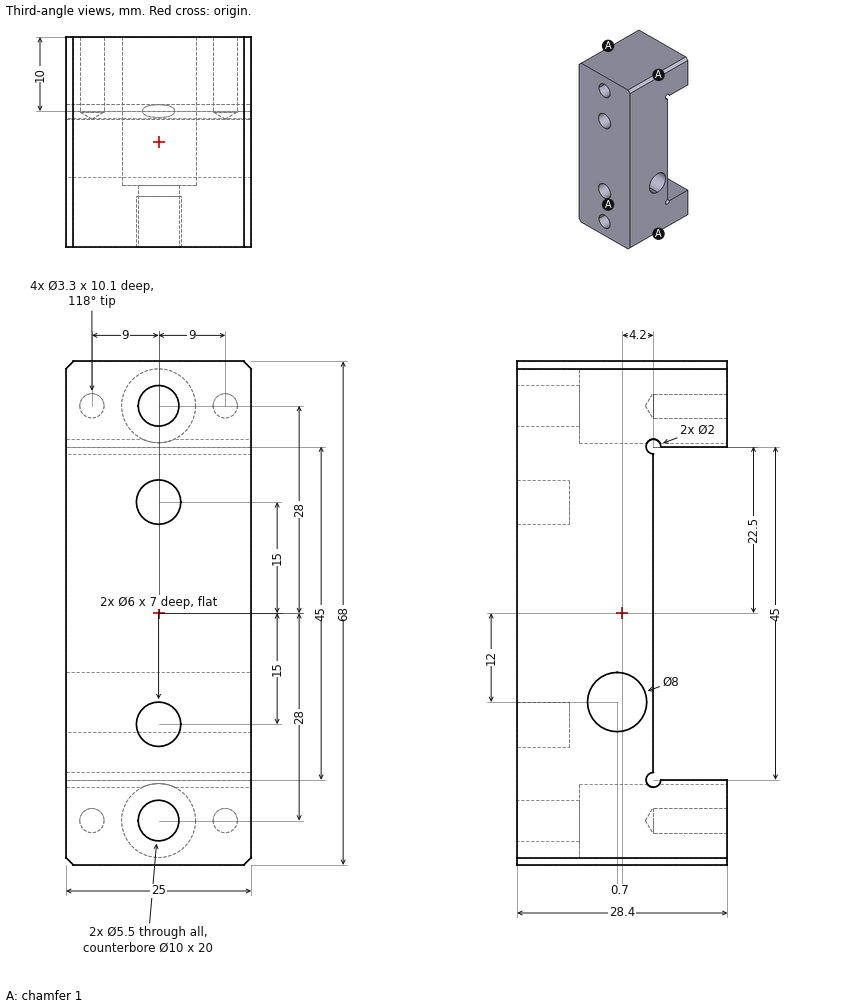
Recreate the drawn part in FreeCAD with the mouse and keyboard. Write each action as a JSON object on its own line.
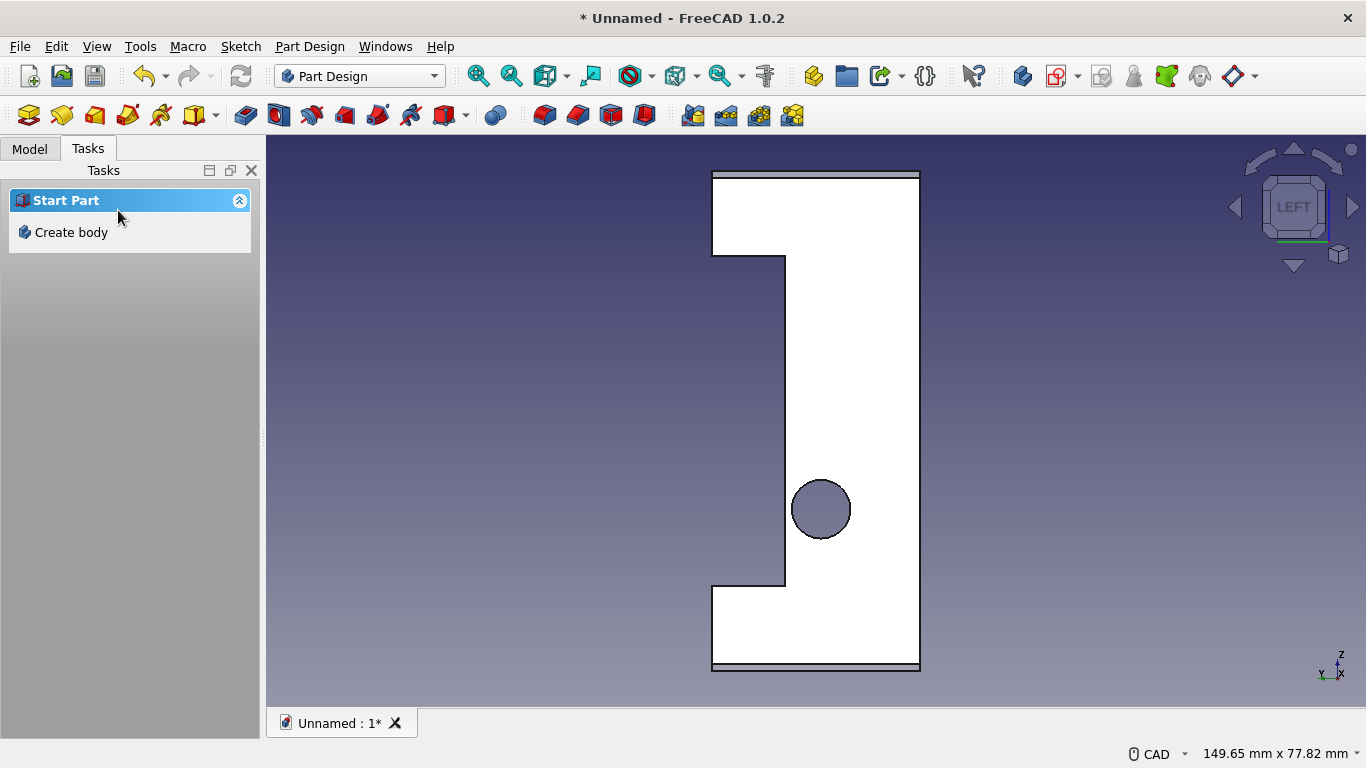
{"action": "key", "text": "0"}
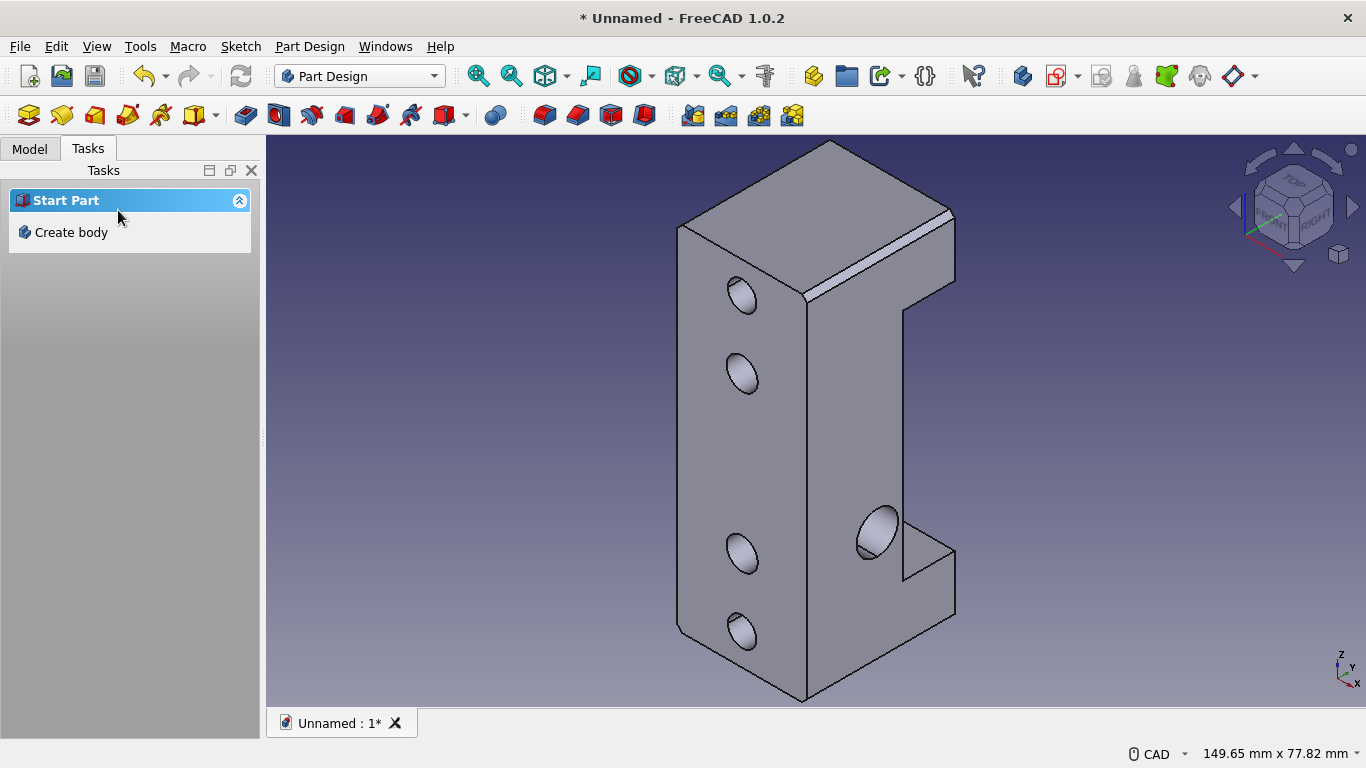
{"action": "left_click", "coordinate": [860, 470]}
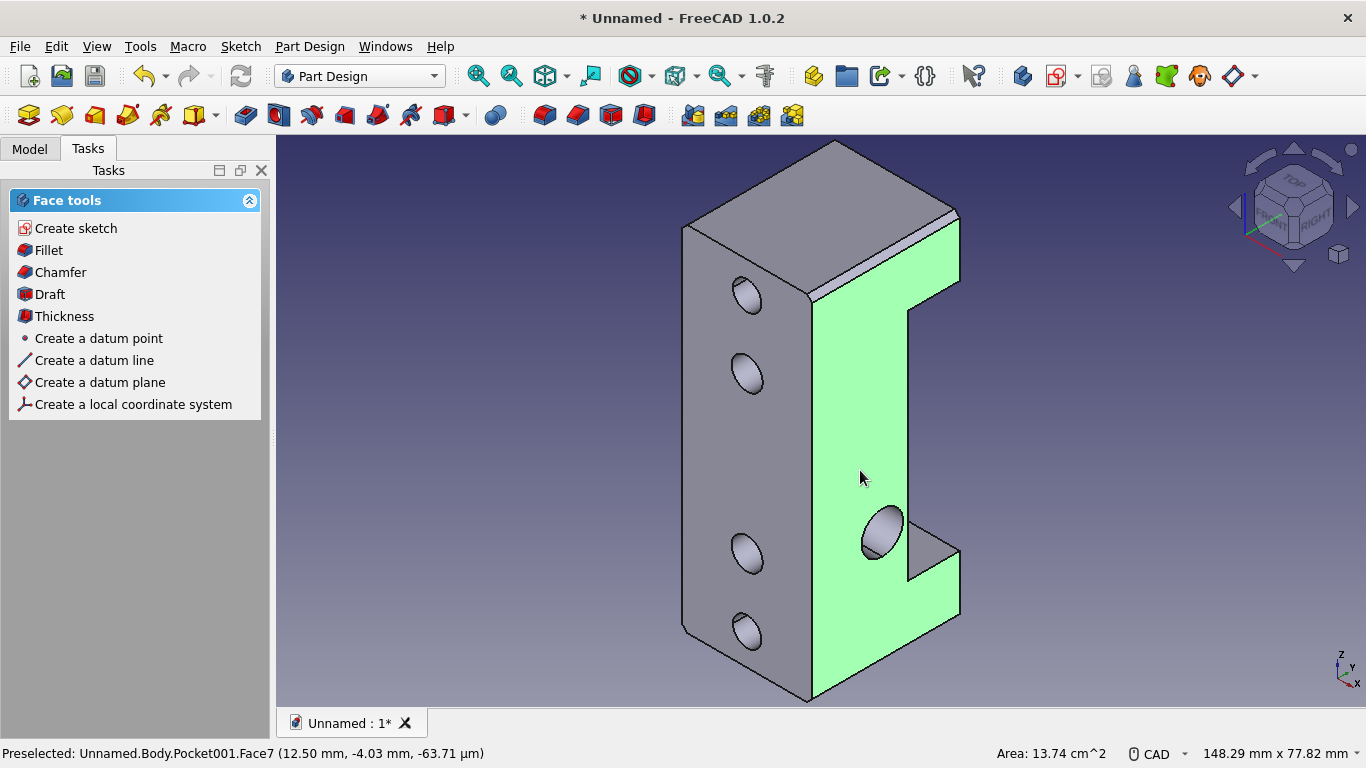
{"action": "left_click", "coordinate": [1056, 76]}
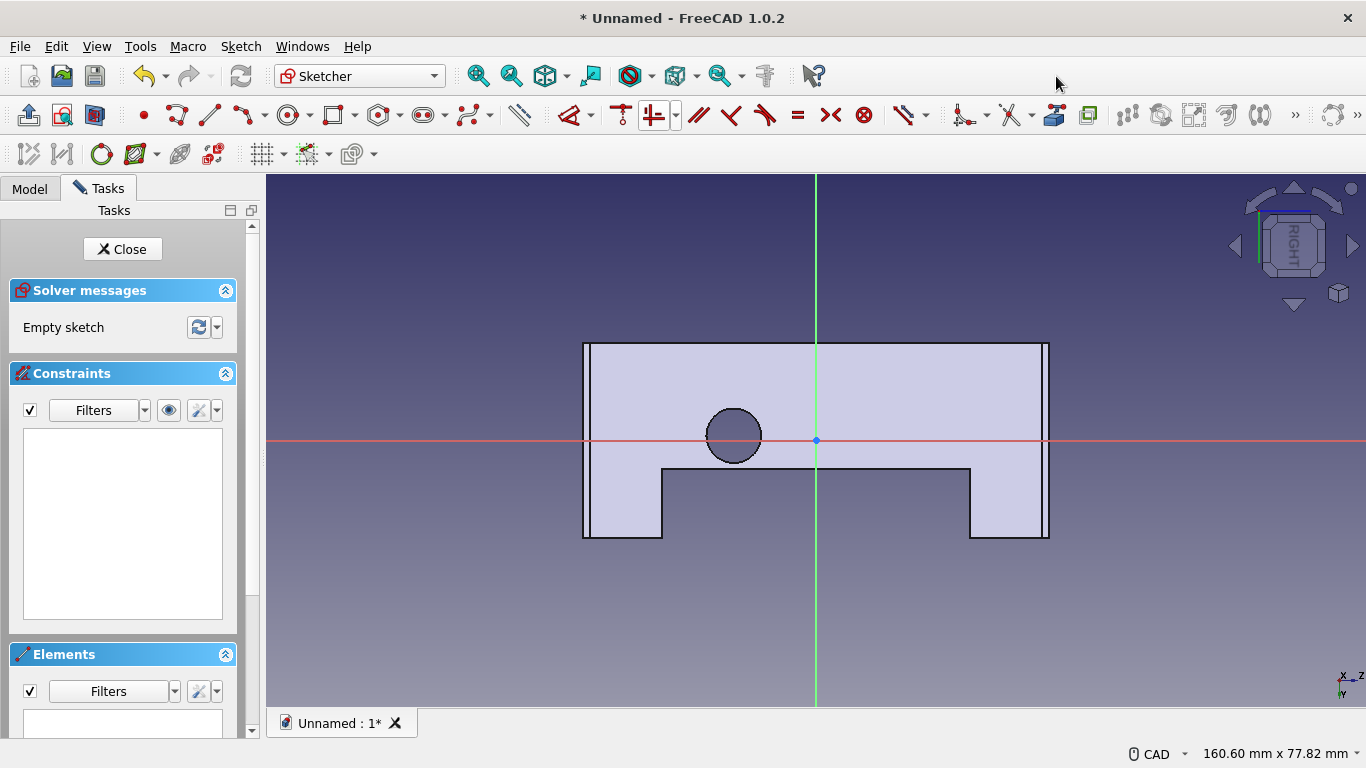
{"action": "scroll", "coordinate": [899, 480], "scroll_direction": "up", "scroll_amount": 3}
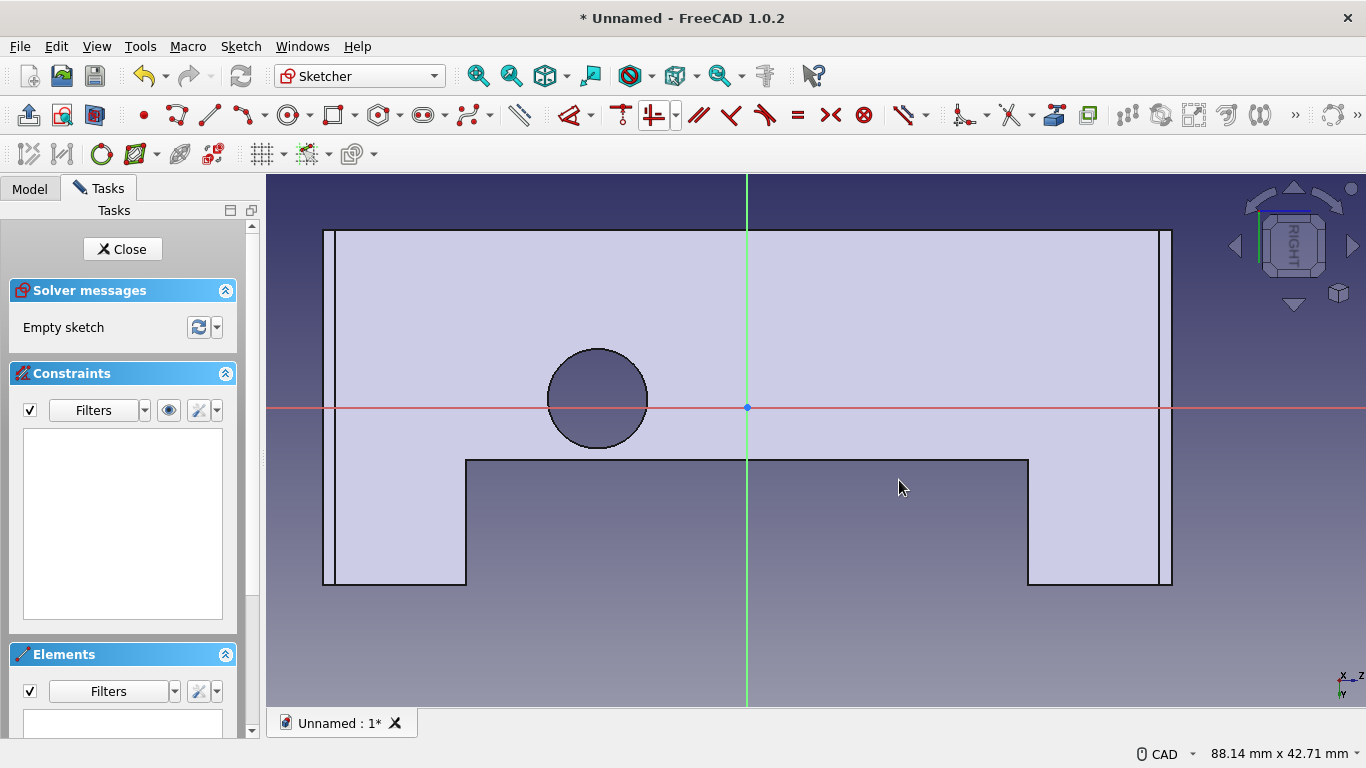
{"action": "key", "text": "g c"}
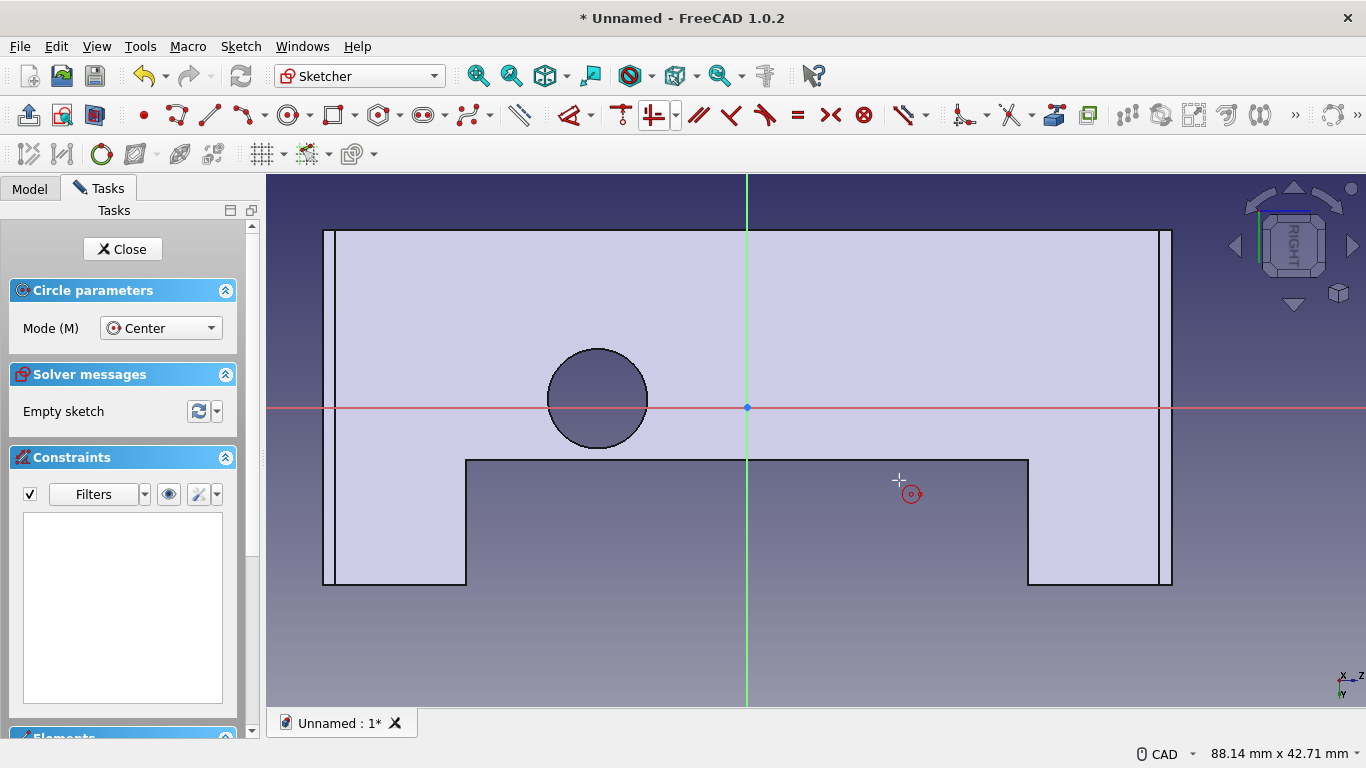
{"action": "scroll", "coordinate": [1028, 460], "scroll_direction": "up", "scroll_amount": 3}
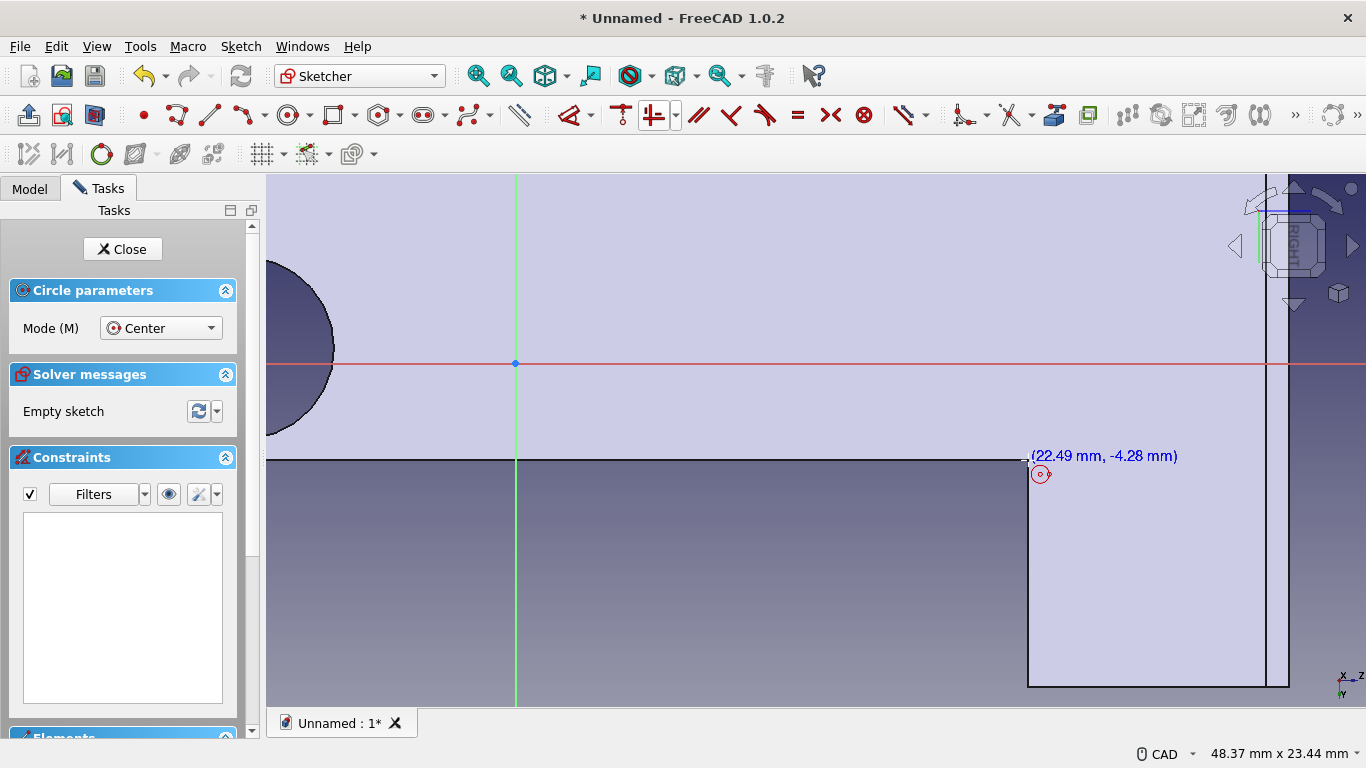
{"action": "left_click", "coordinate": [1028, 460]}
{"action": "left_click", "coordinate": [1044, 443]}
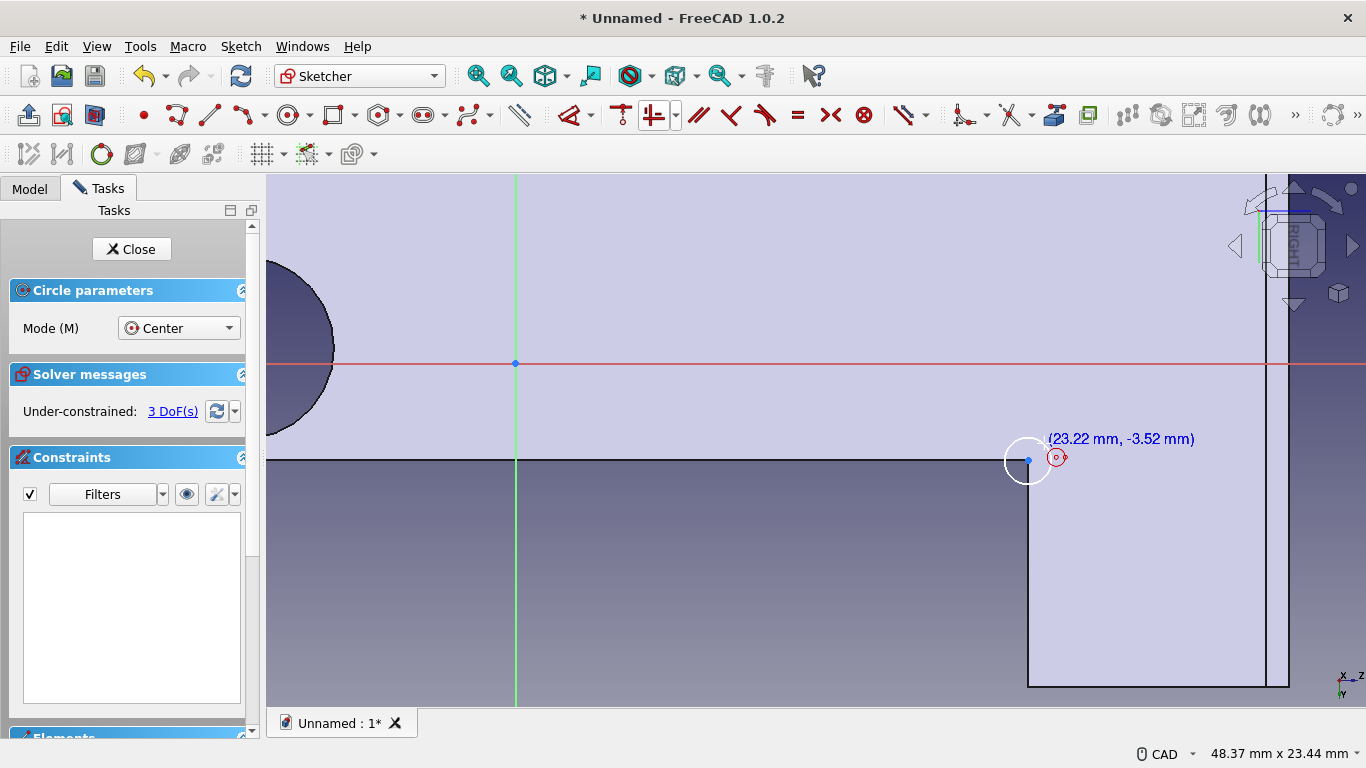
{"action": "scroll", "coordinate": [1029, 462], "scroll_direction": "down", "scroll_amount": 3}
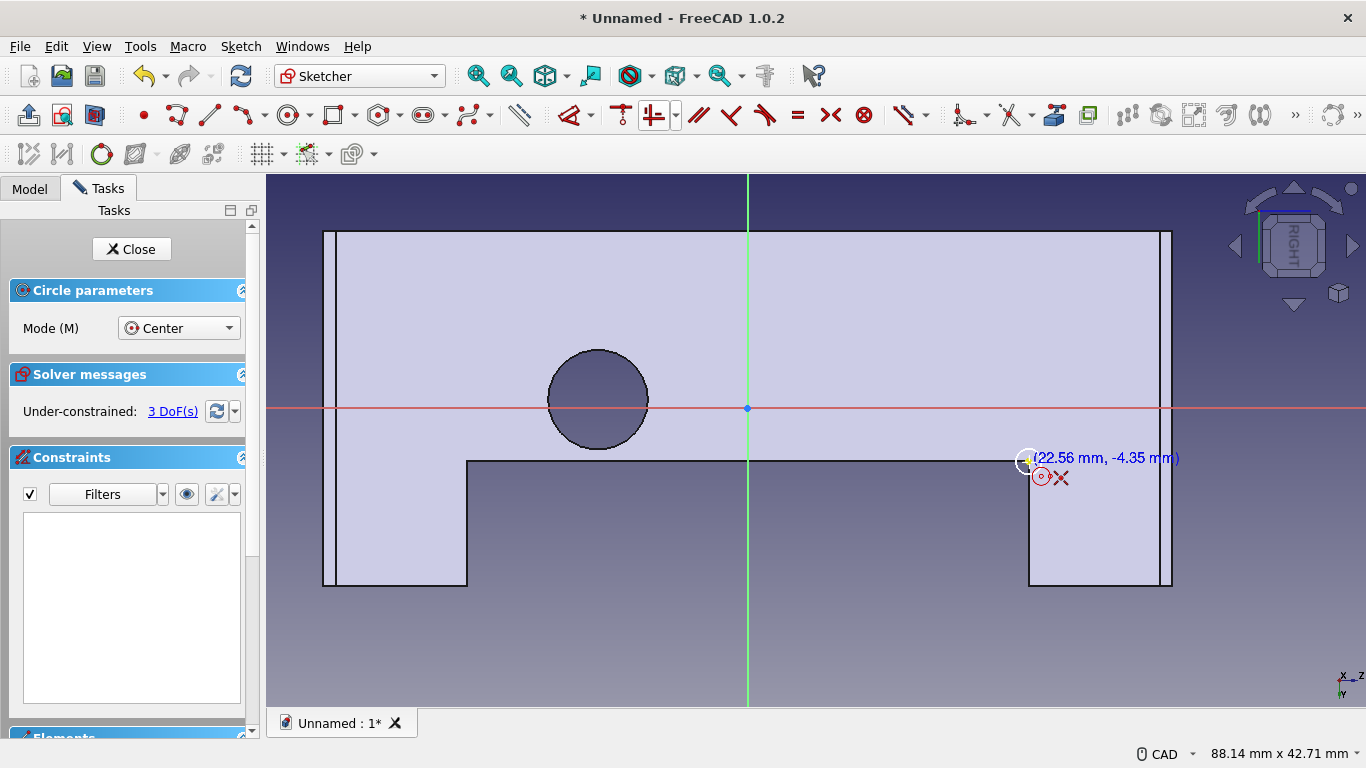
{"action": "scroll", "coordinate": [467, 461], "scroll_direction": "up", "scroll_amount": 3}